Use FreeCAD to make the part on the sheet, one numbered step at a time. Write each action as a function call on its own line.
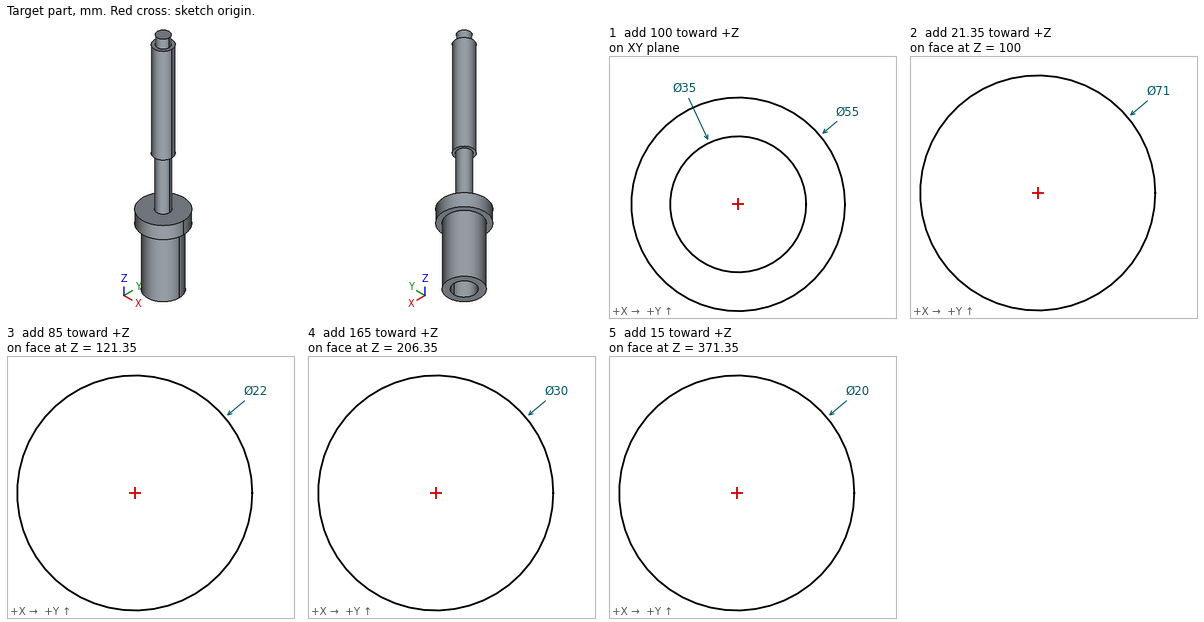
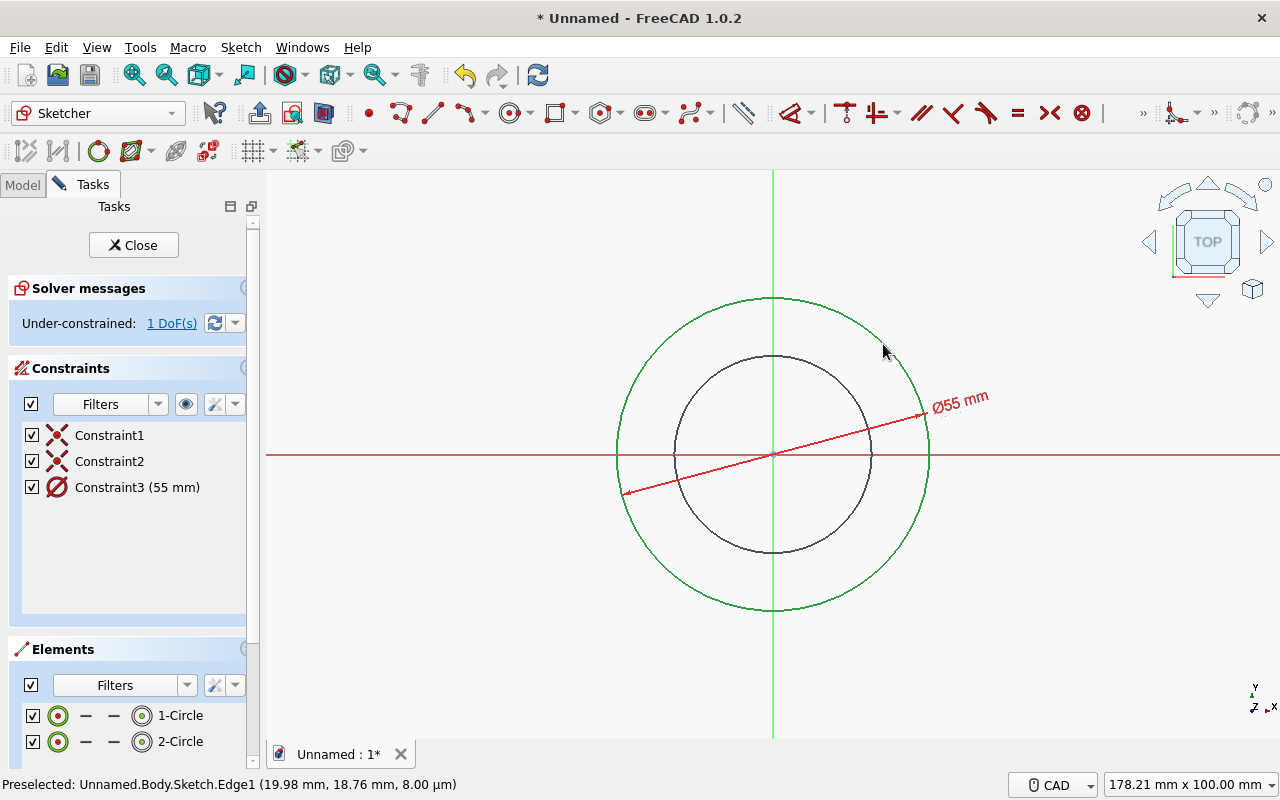
click(843, 385)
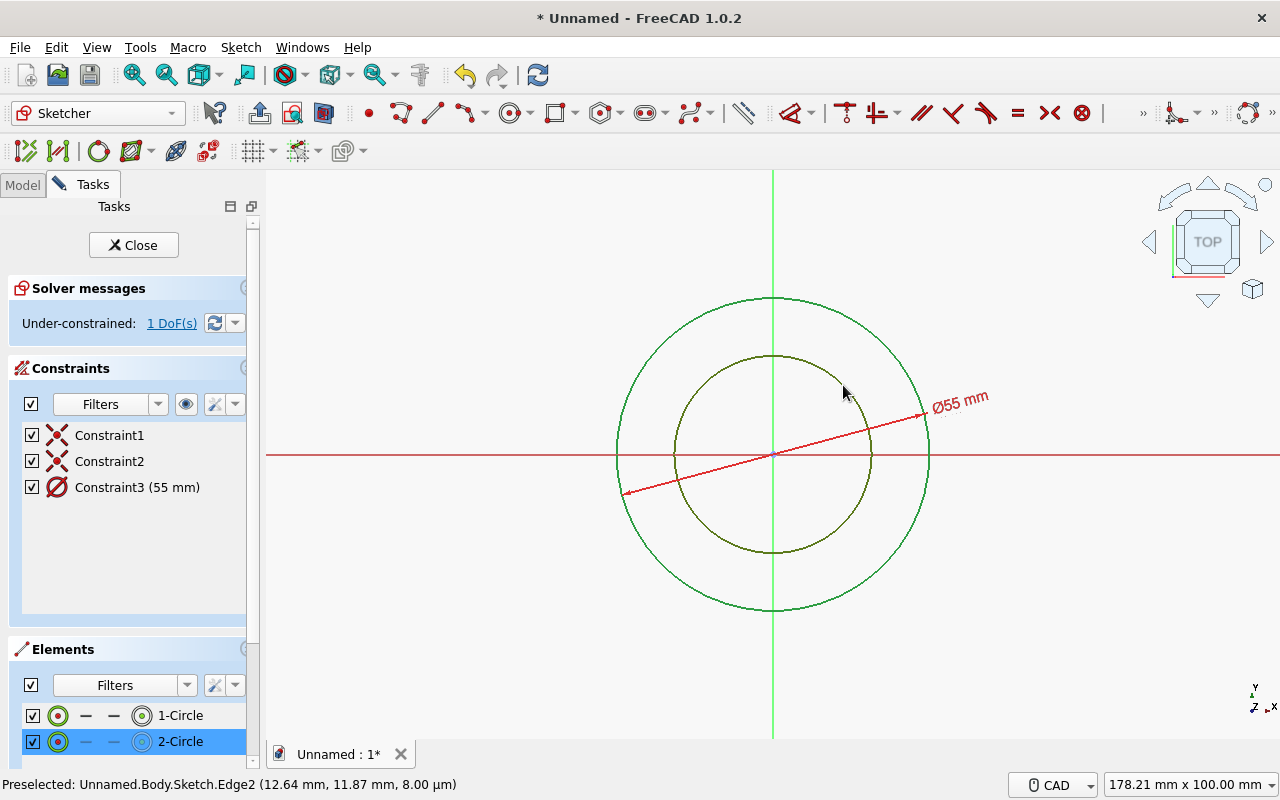
key(k)
key(o)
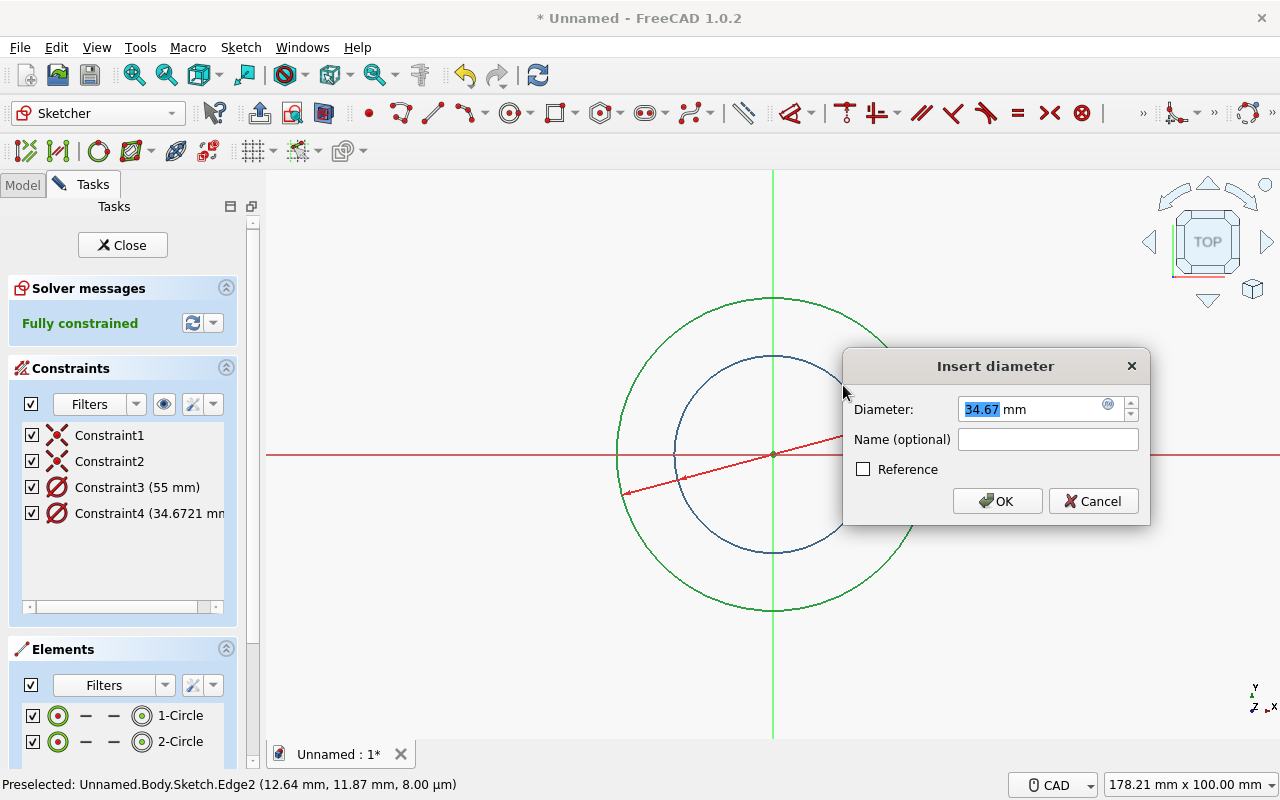
text(35)
key(Return)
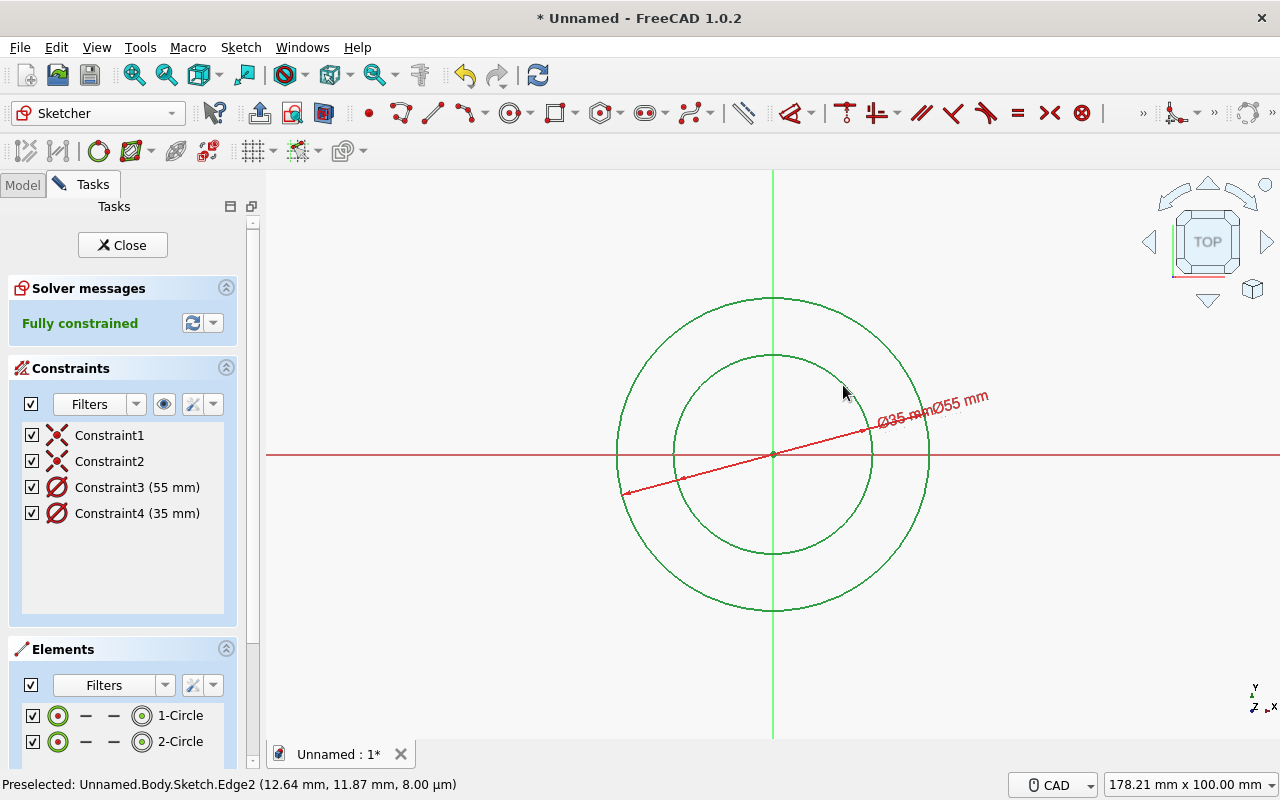
click(123, 245)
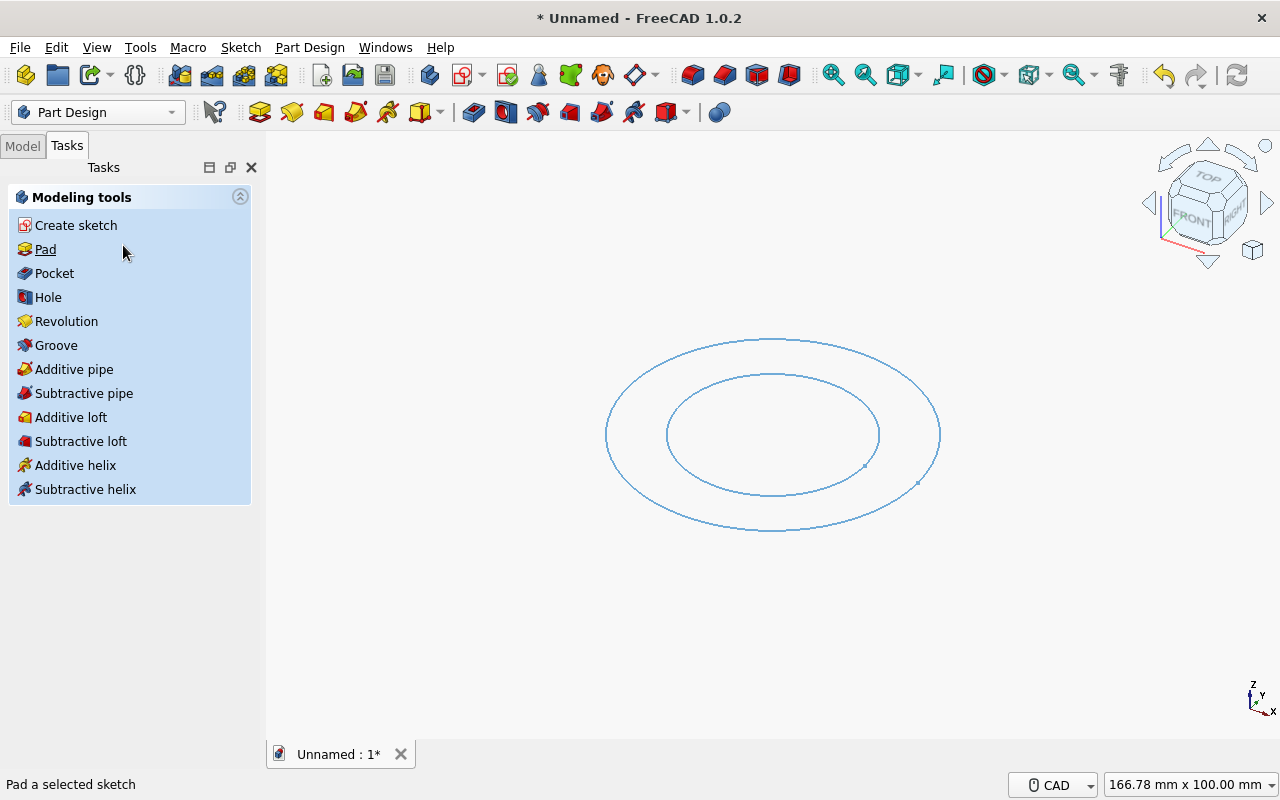
click(260, 112)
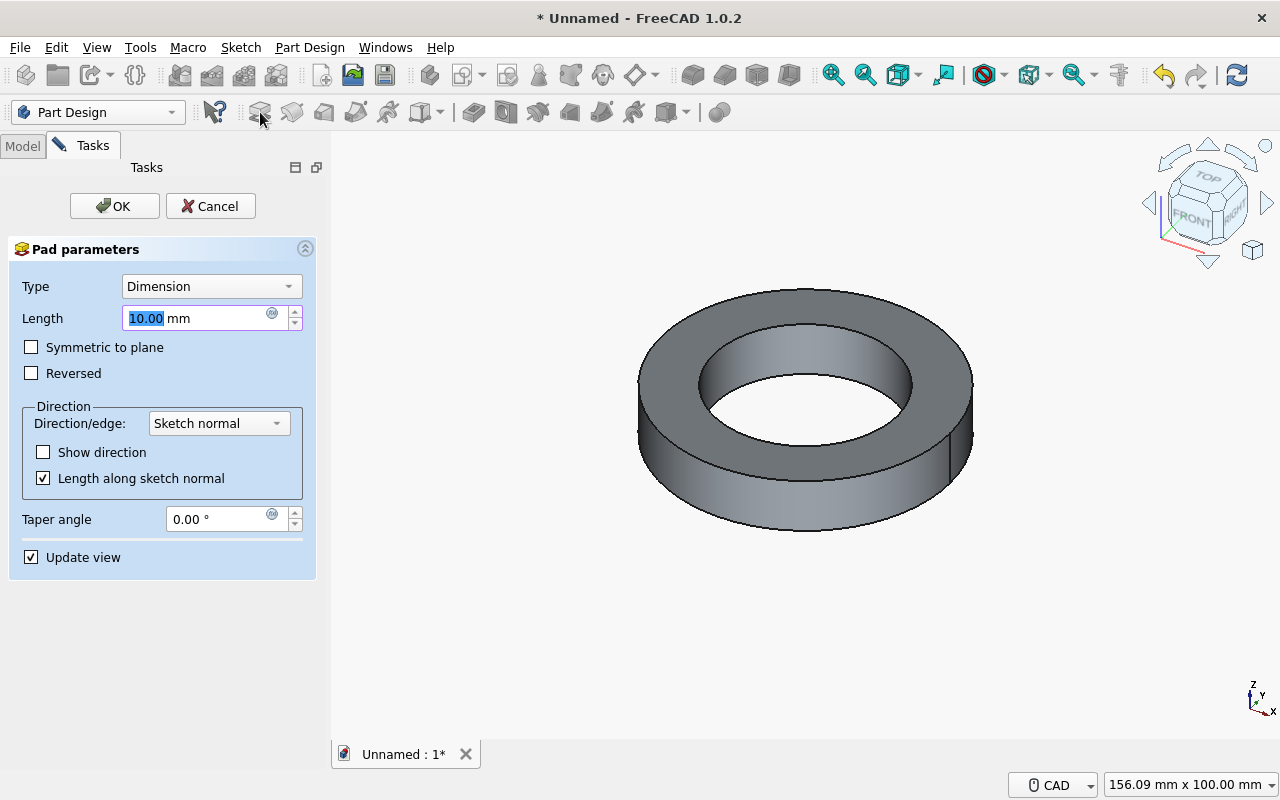
text(100)
key(Tab)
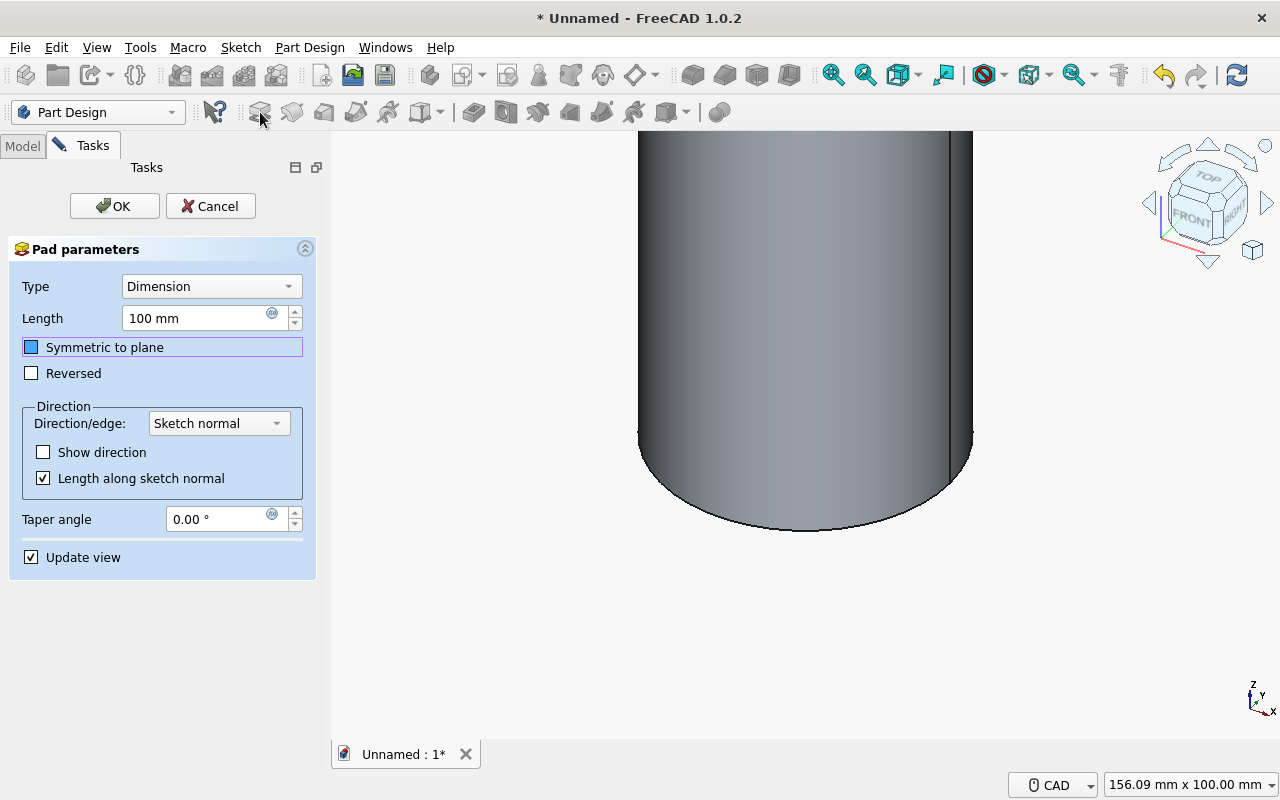
click(115, 206)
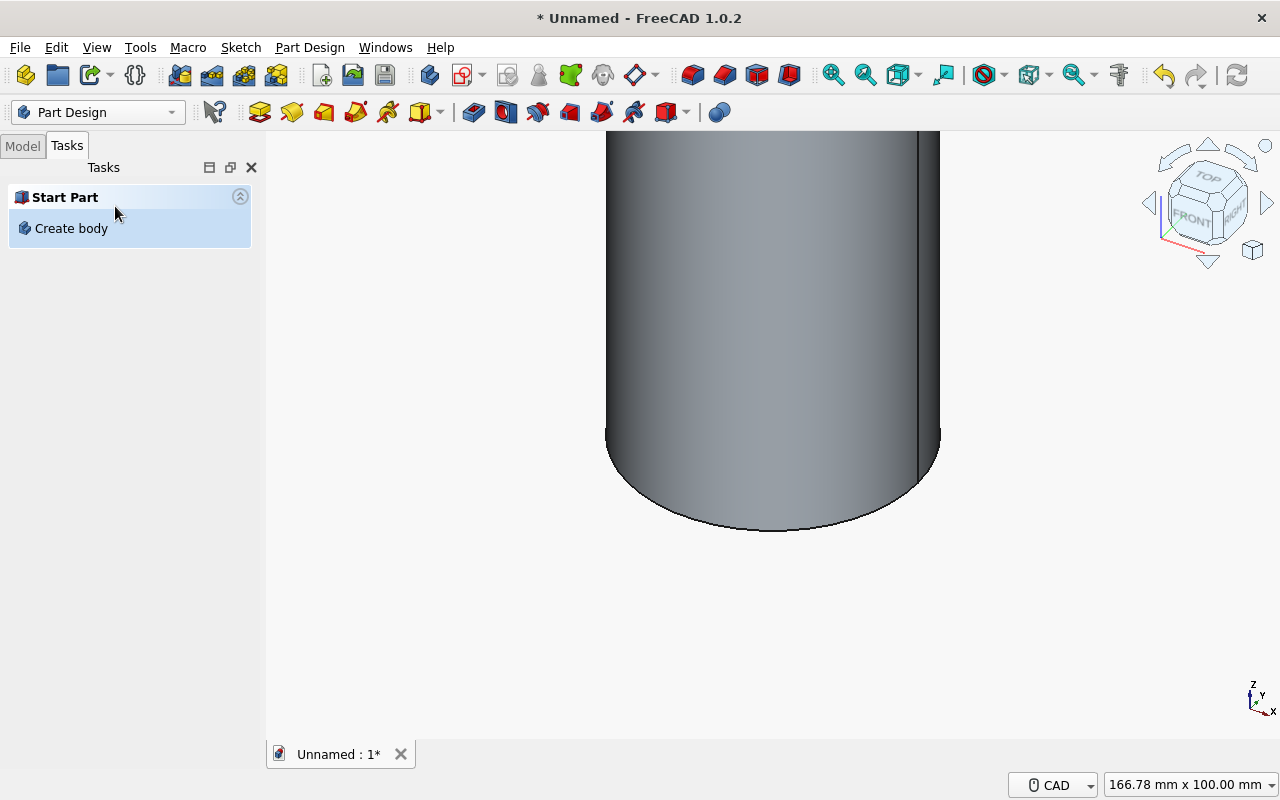
click(834, 76)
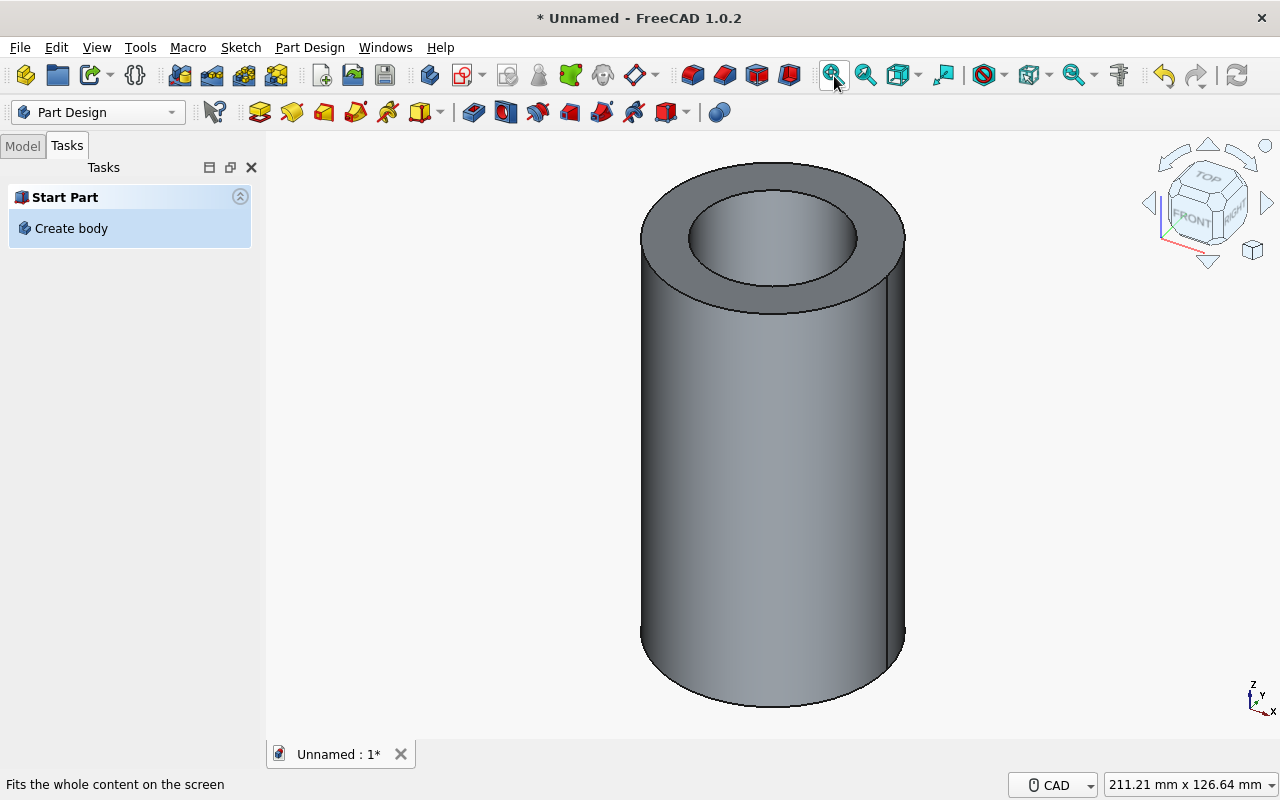
click(745, 178)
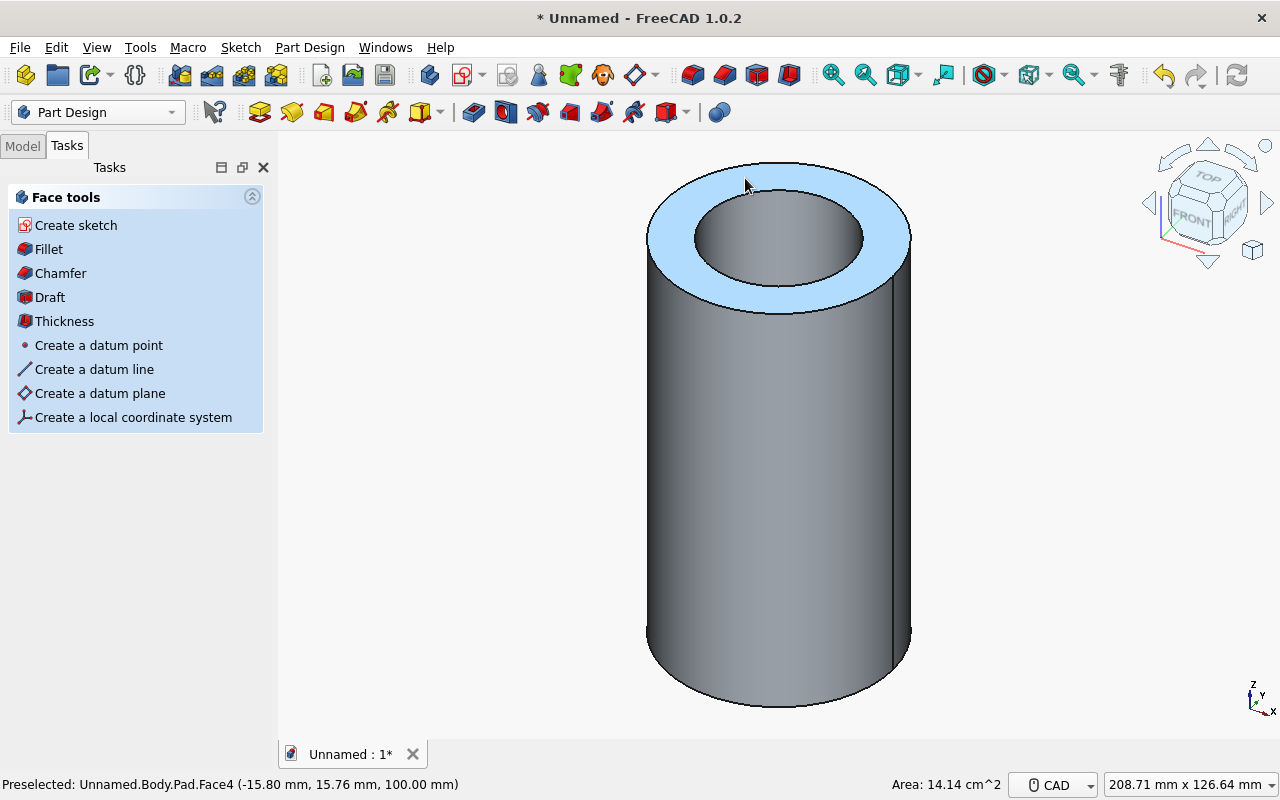
click(462, 76)